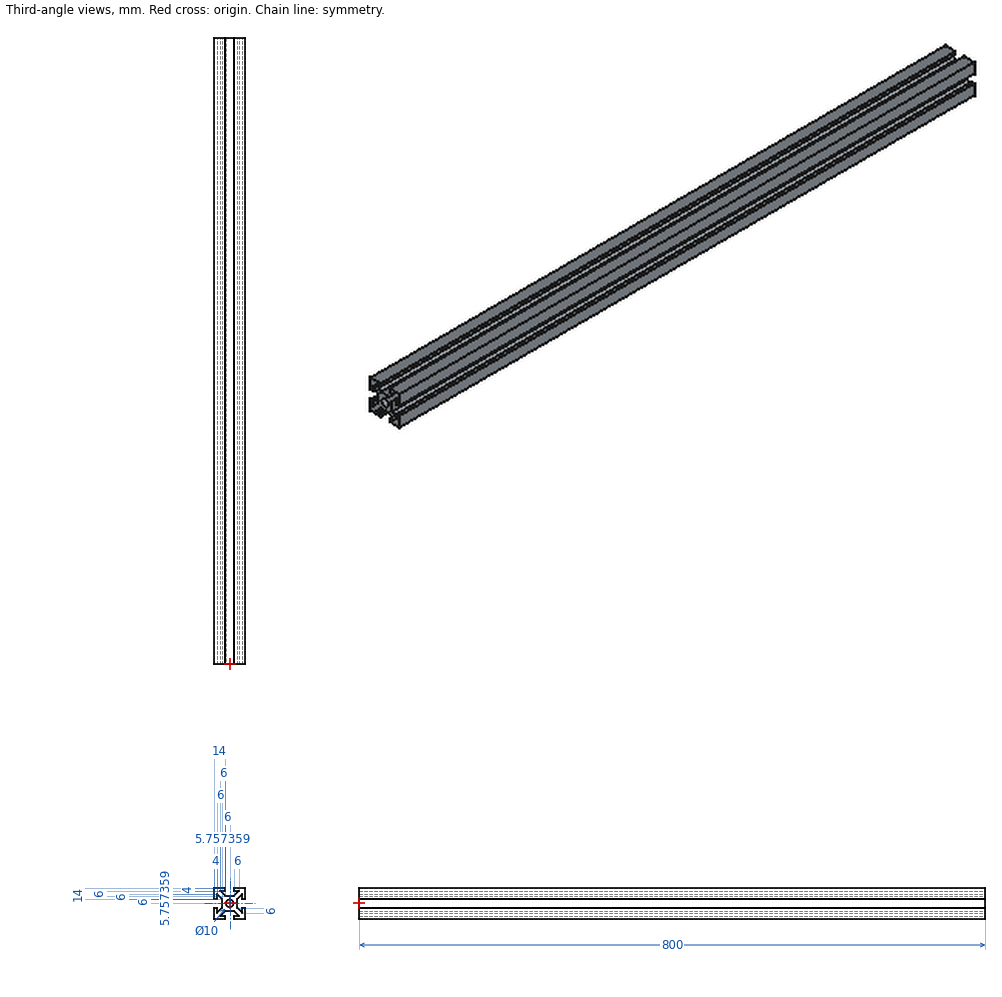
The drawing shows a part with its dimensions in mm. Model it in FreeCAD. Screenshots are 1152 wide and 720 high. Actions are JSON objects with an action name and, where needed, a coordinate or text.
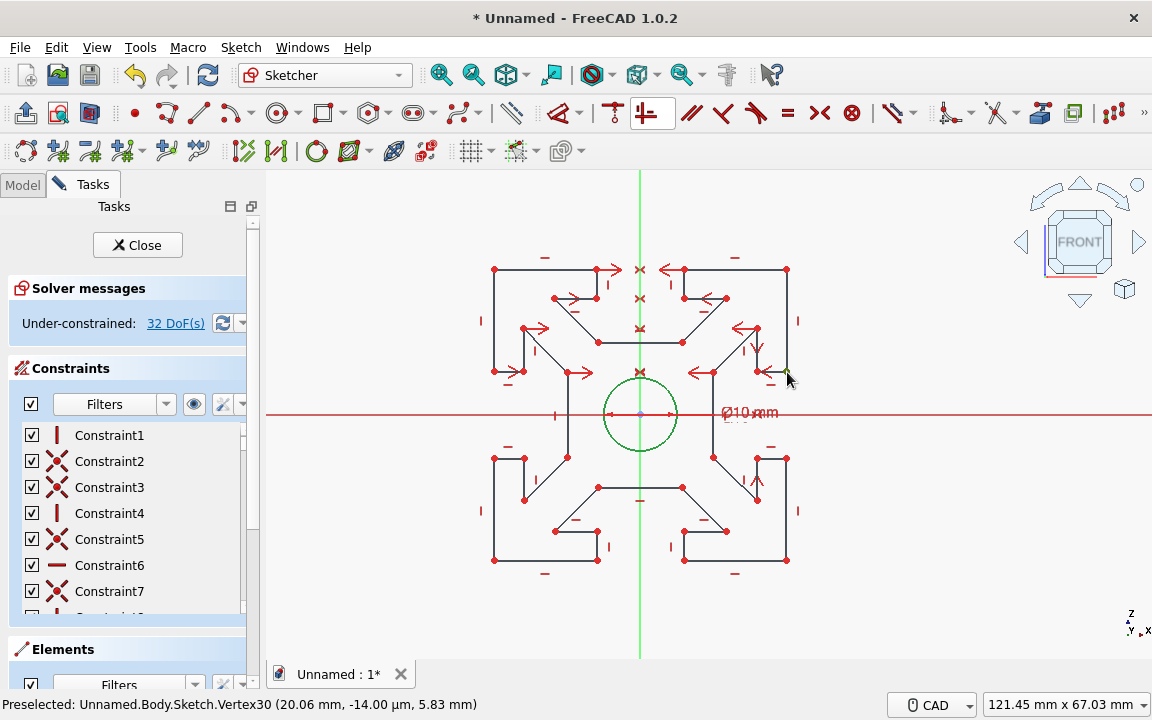
{"action": "left_click", "coordinate": [786, 459]}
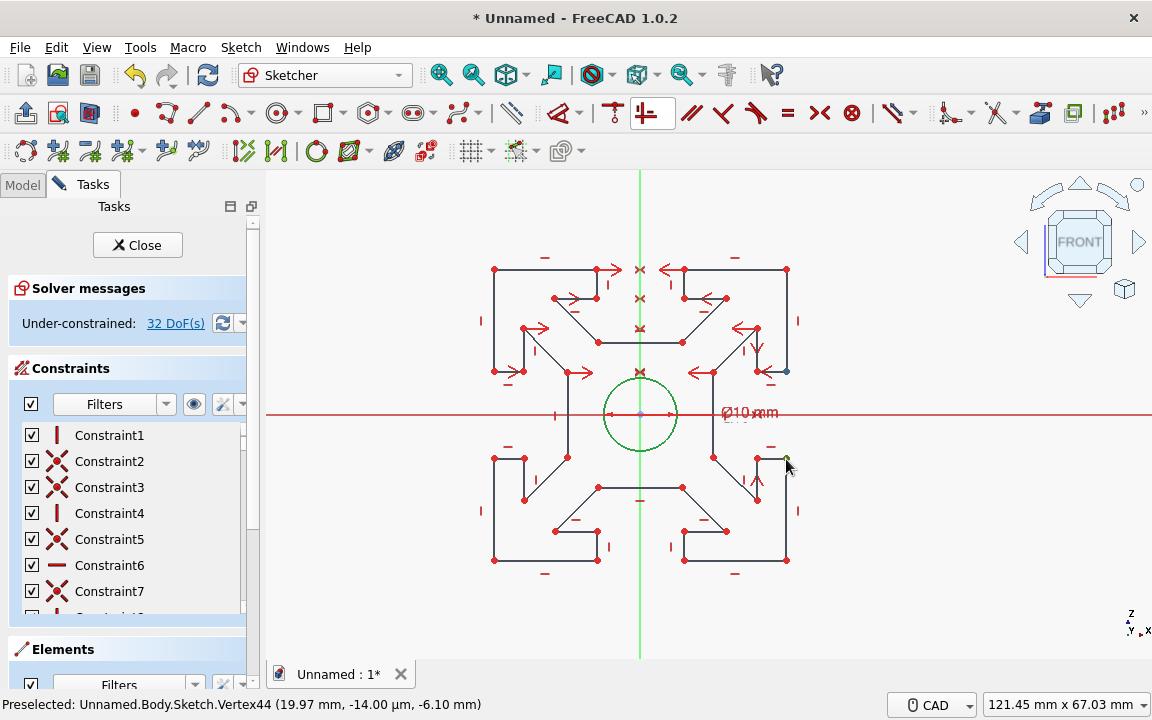
{"action": "left_click", "coordinate": [344, 414]}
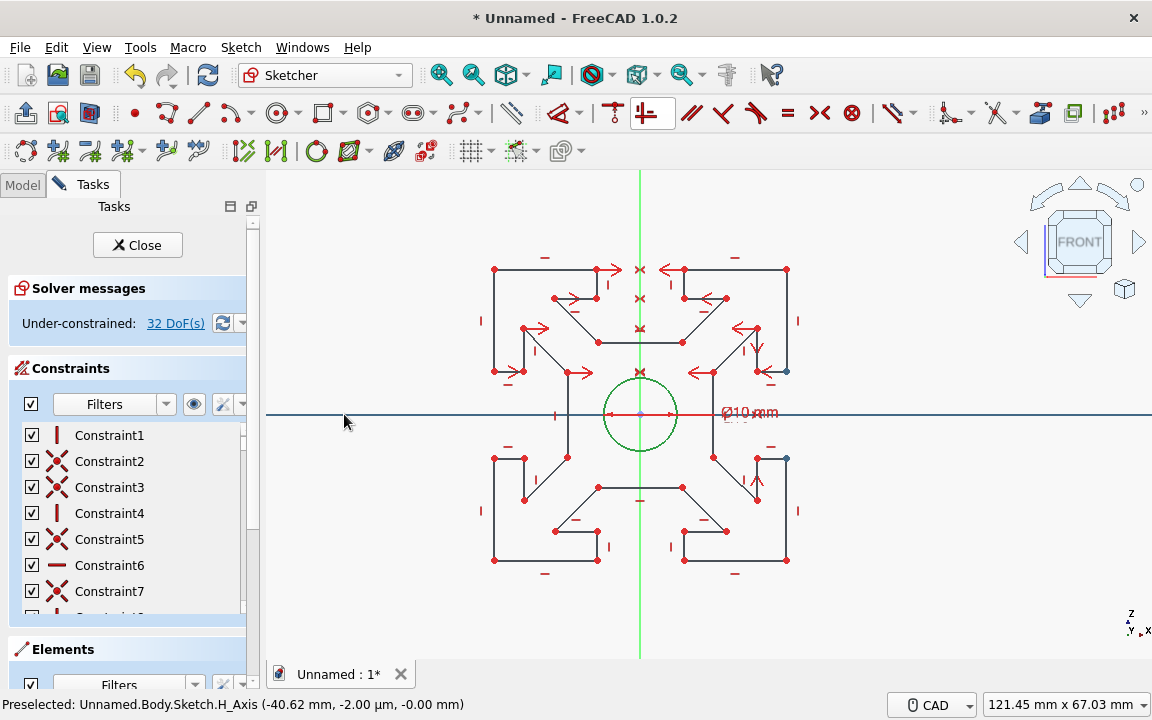
{"action": "key", "text": "s"}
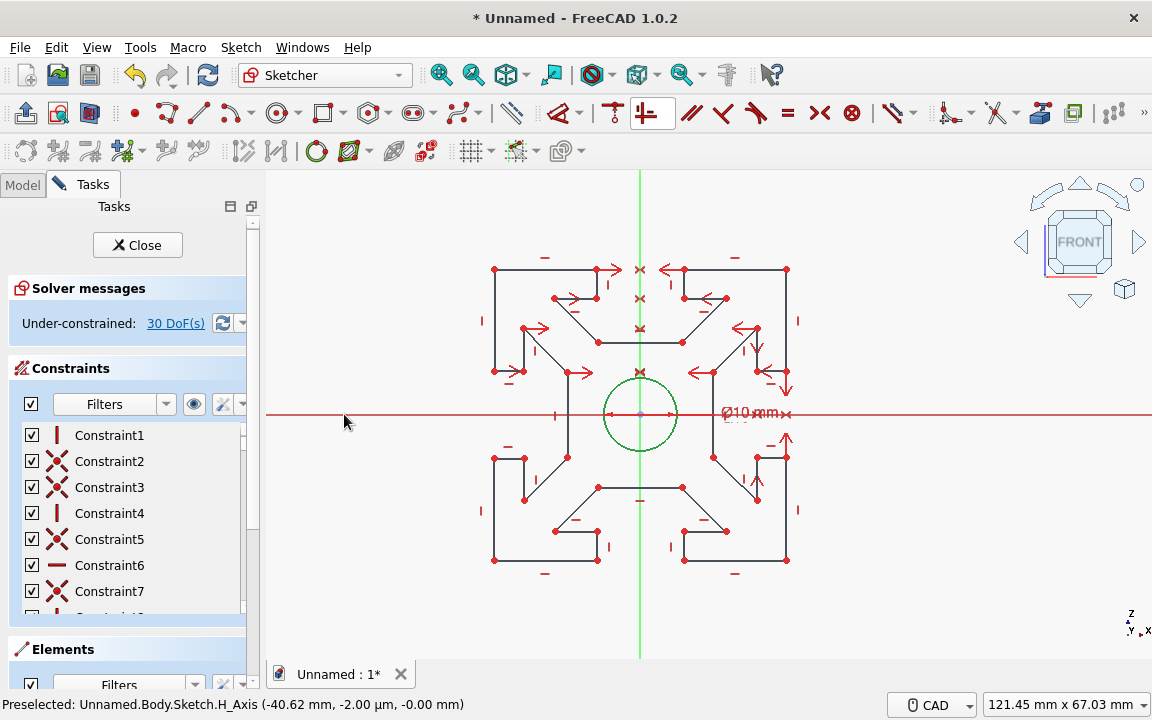
{"action": "left_click", "coordinate": [684, 270]}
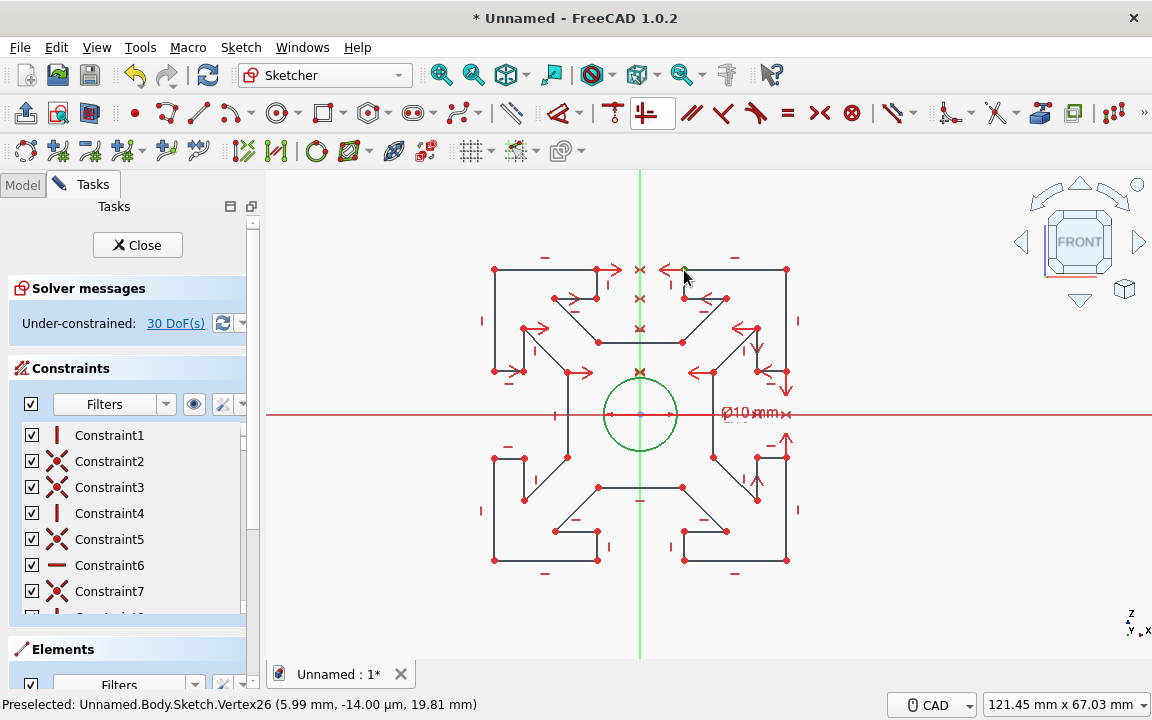
{"action": "left_click", "coordinate": [684, 561]}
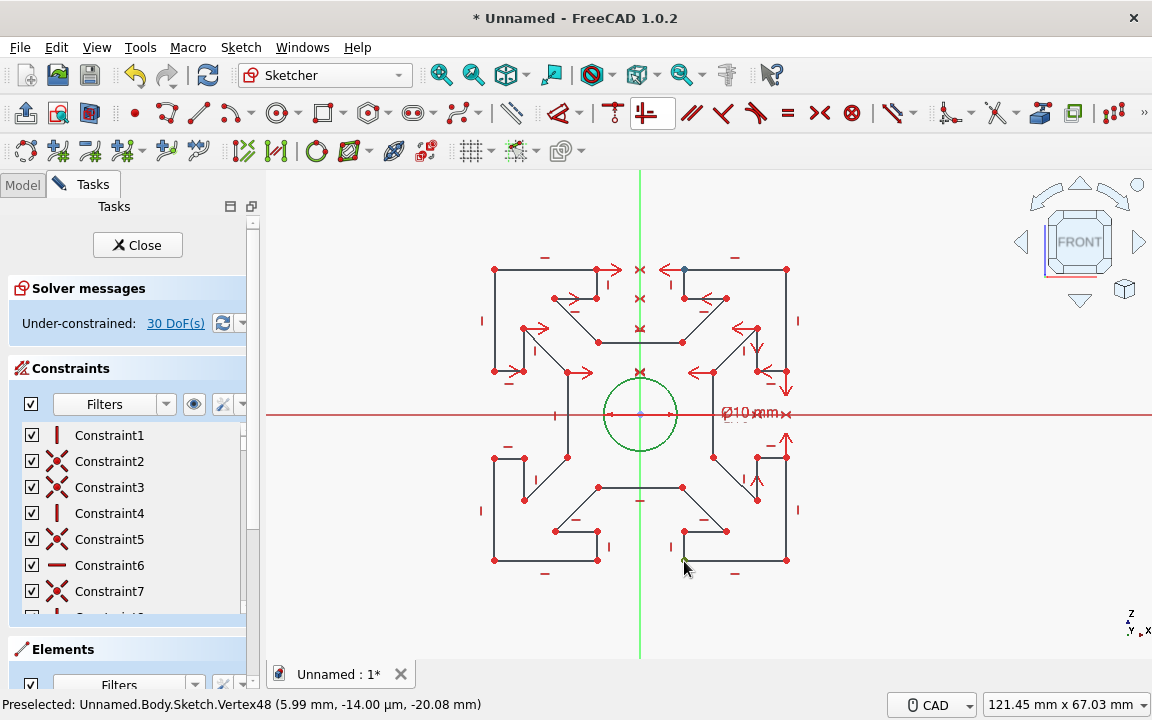
{"action": "left_click", "coordinate": [344, 414]}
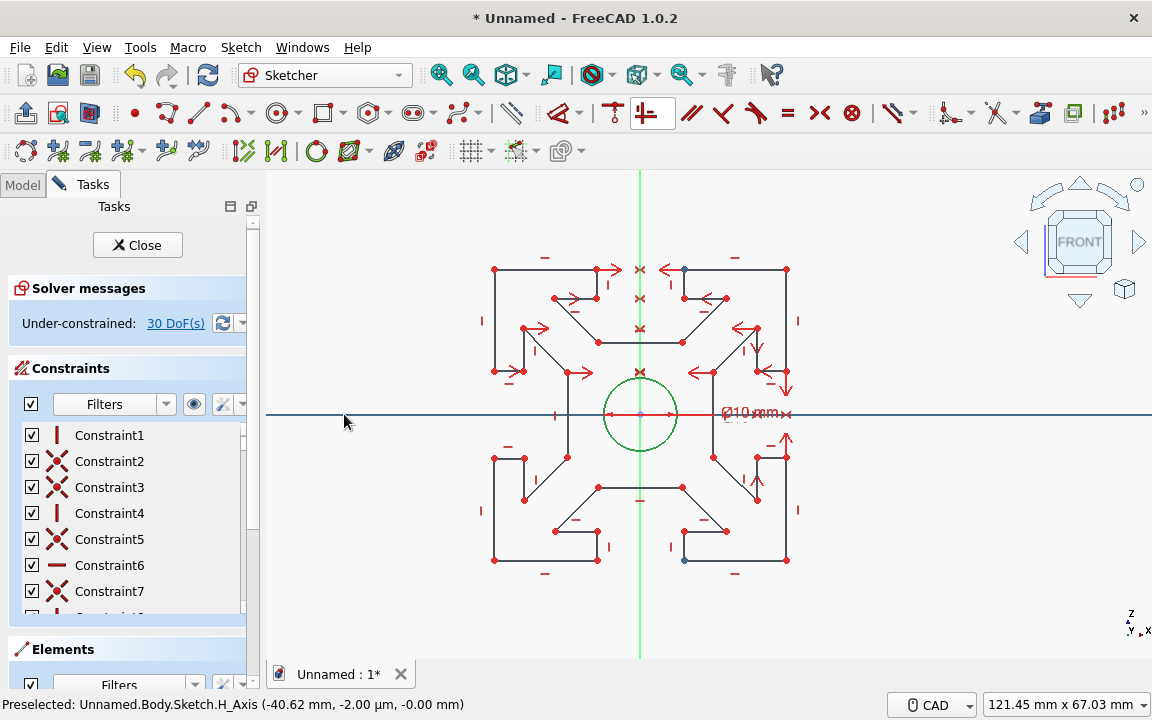
{"action": "key", "text": "s"}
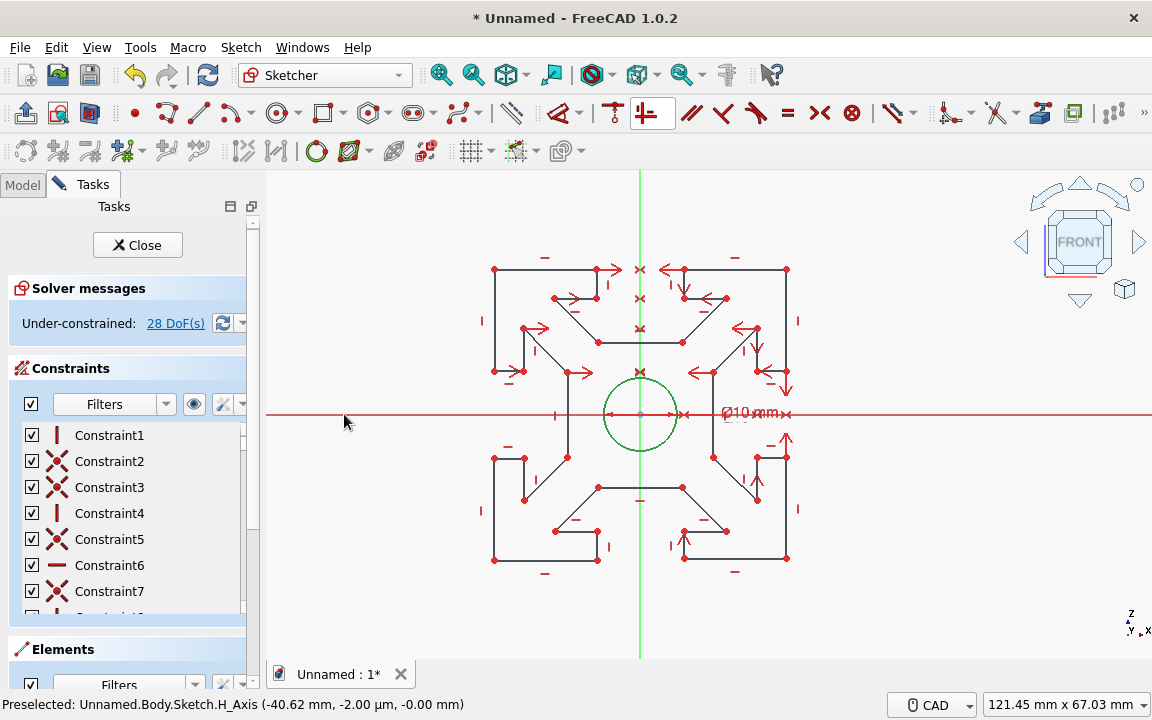
{"action": "left_click", "coordinate": [726, 299]}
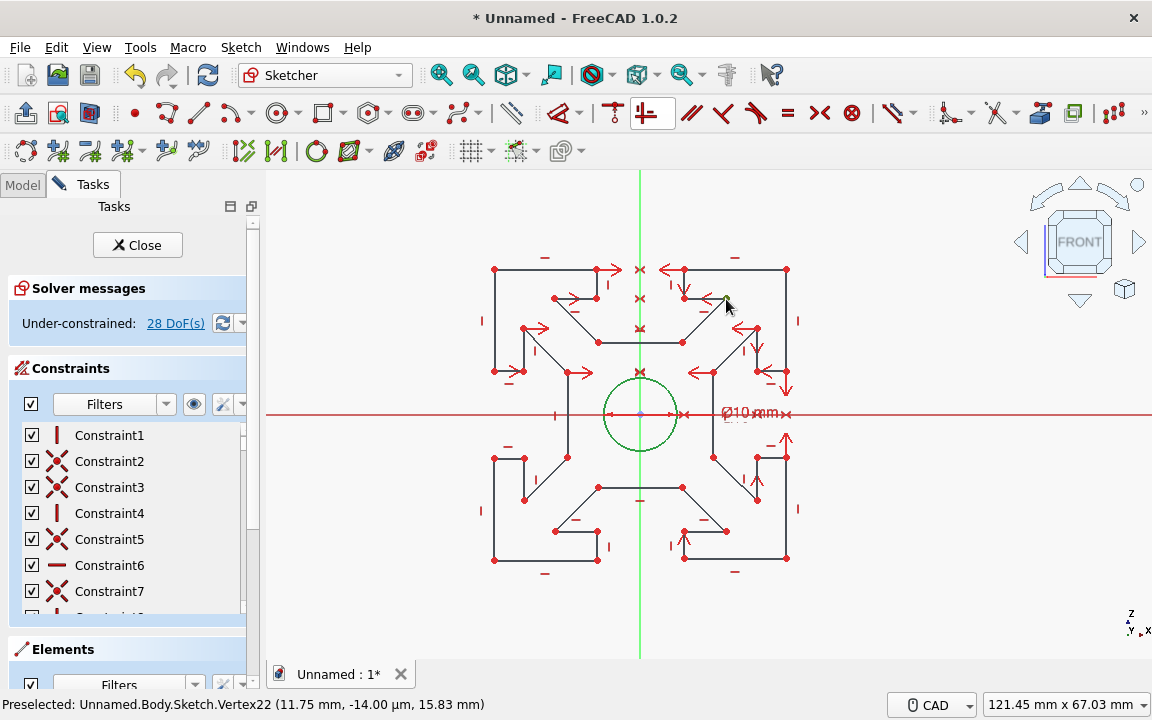
{"action": "left_click", "coordinate": [726, 532]}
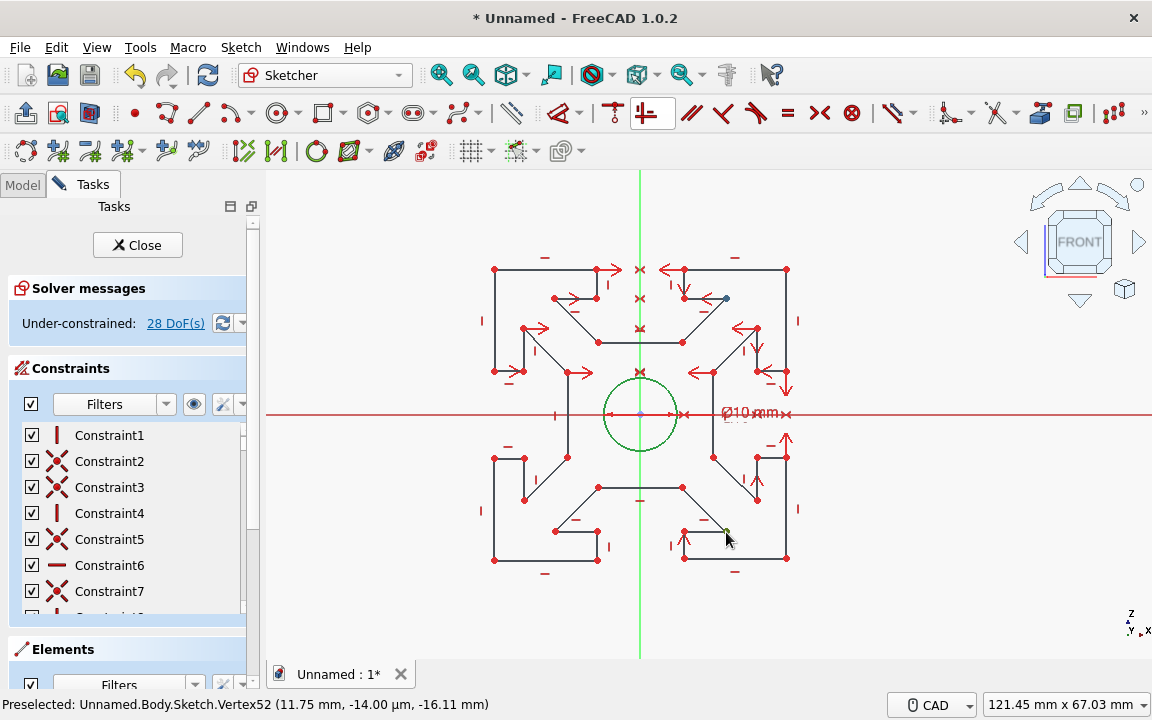
{"action": "left_click", "coordinate": [344, 414]}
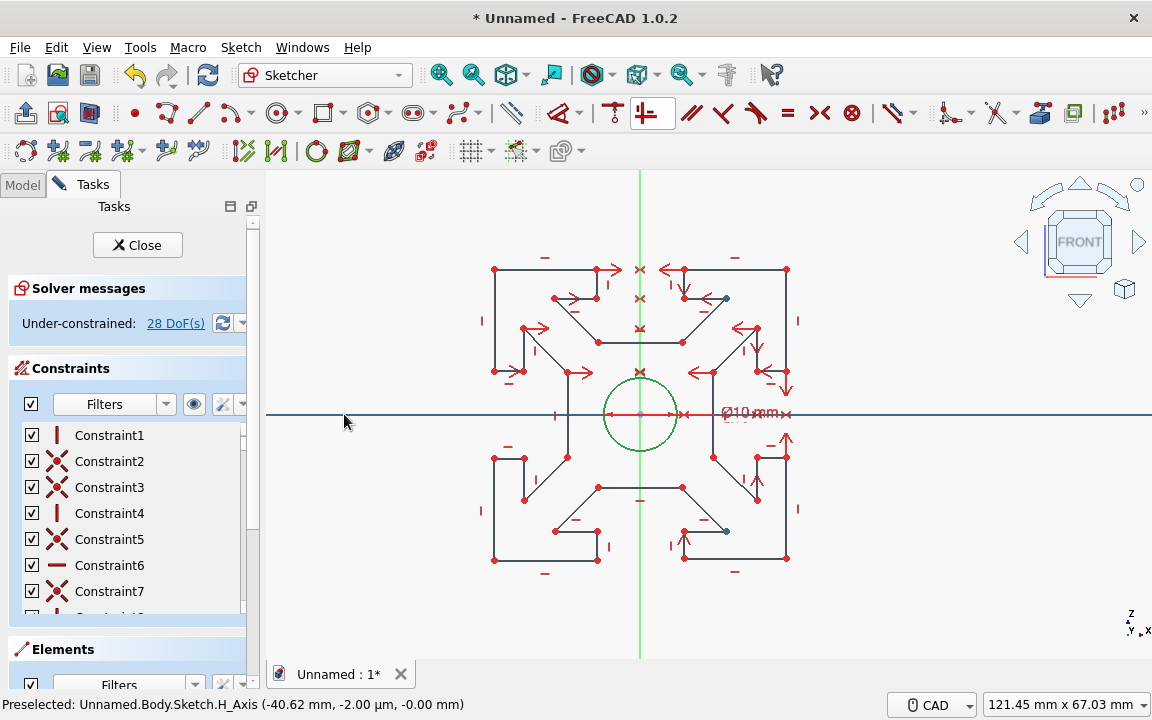
{"action": "key", "text": "s"}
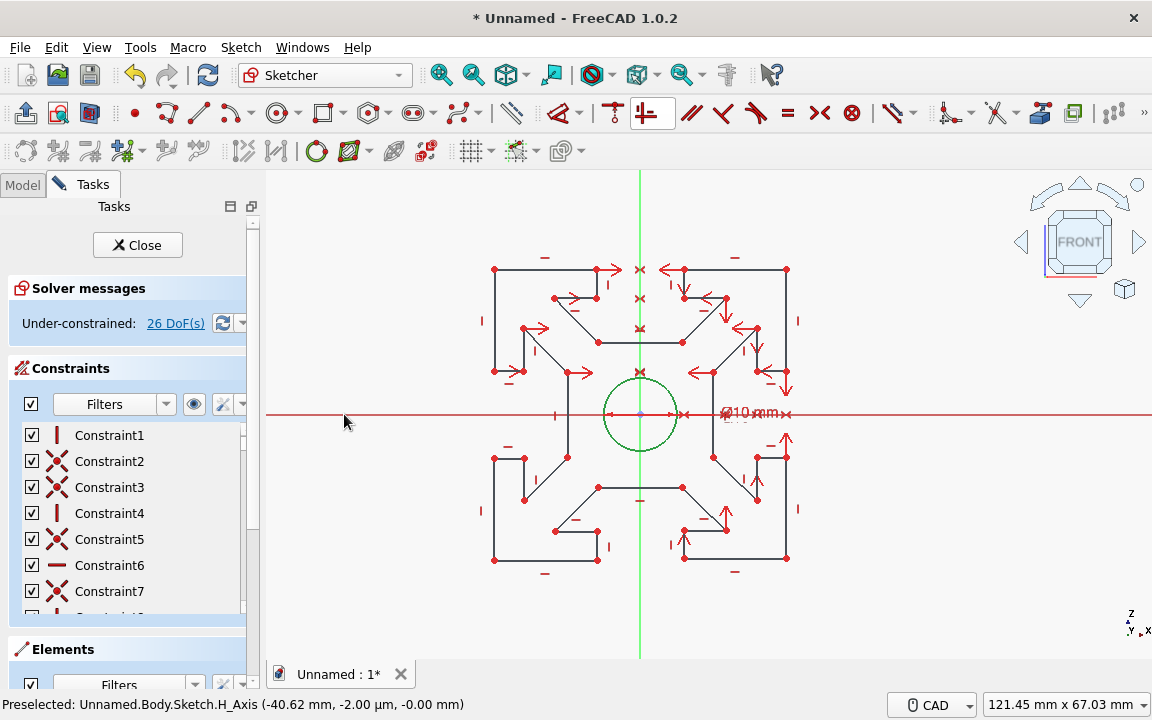
{"action": "left_click", "coordinate": [682, 343]}